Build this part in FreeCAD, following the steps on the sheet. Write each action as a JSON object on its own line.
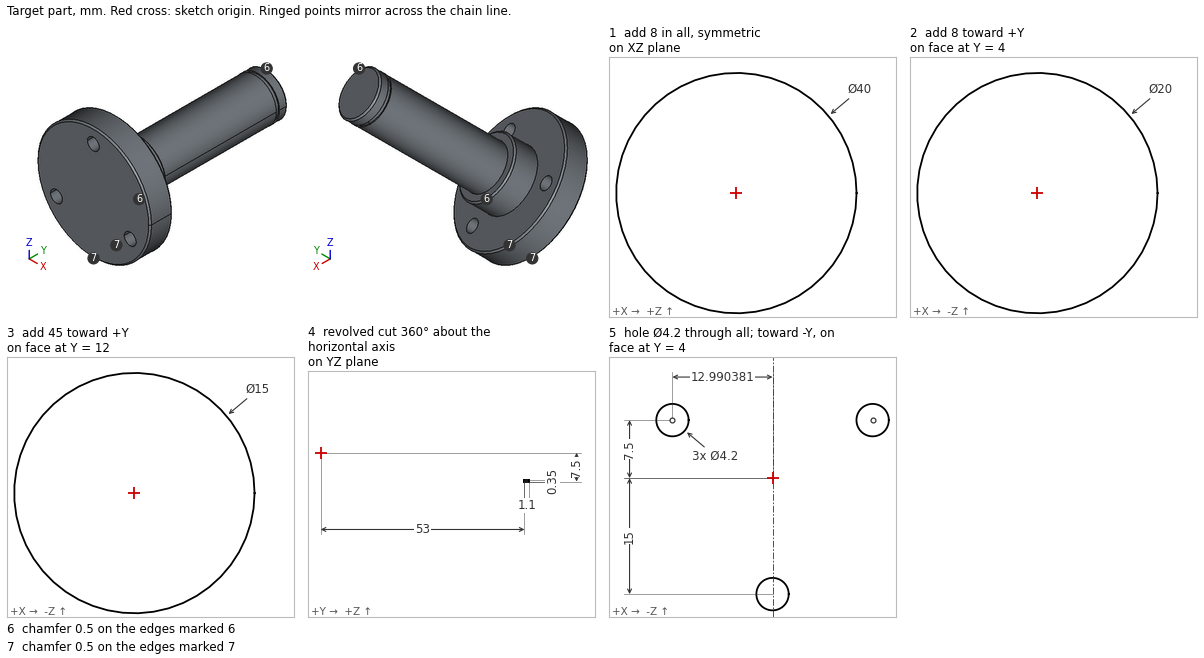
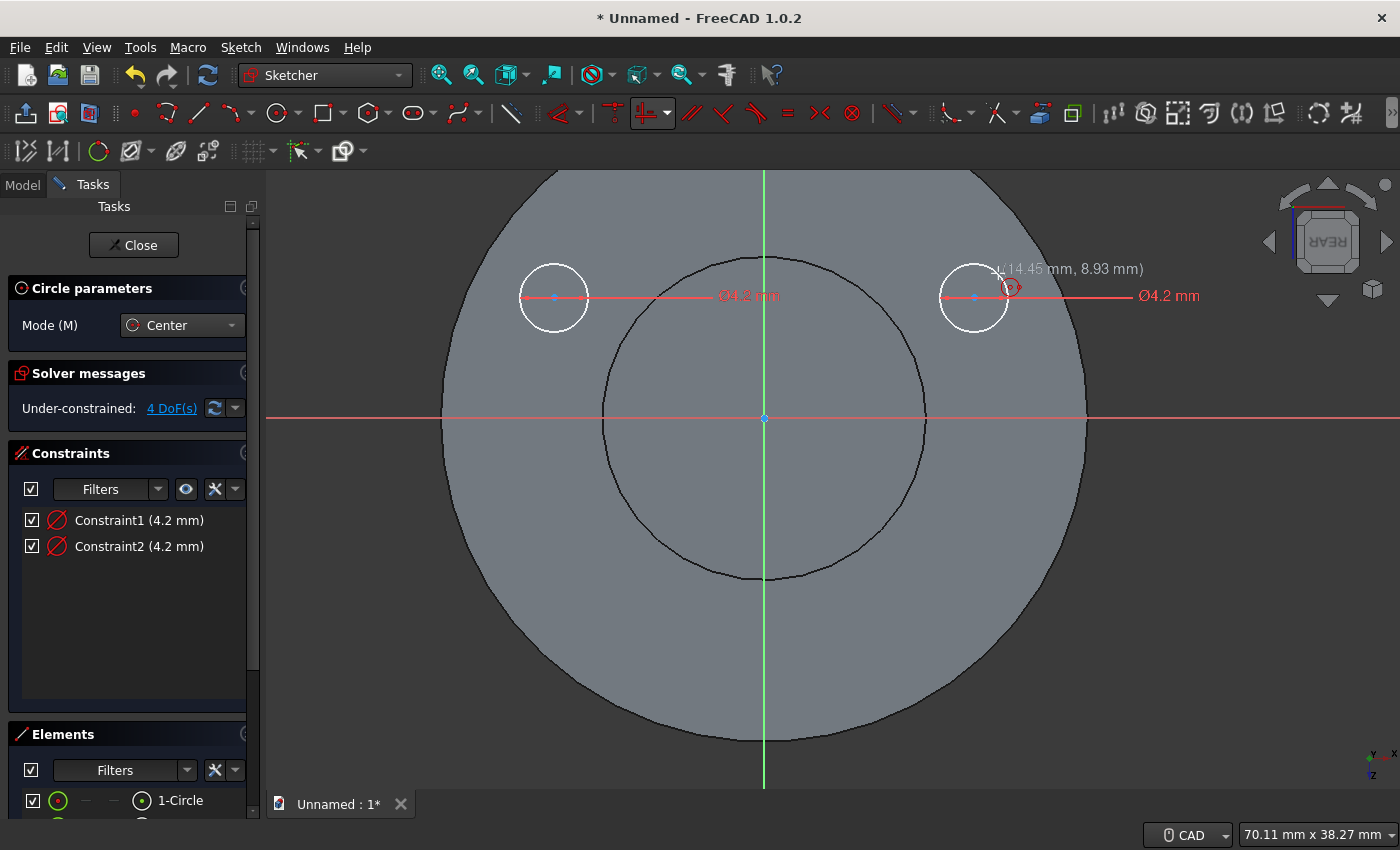
{"action": "left_click", "coordinate": [764, 661]}
{"action": "mouse_move", "coordinate": [788, 637]}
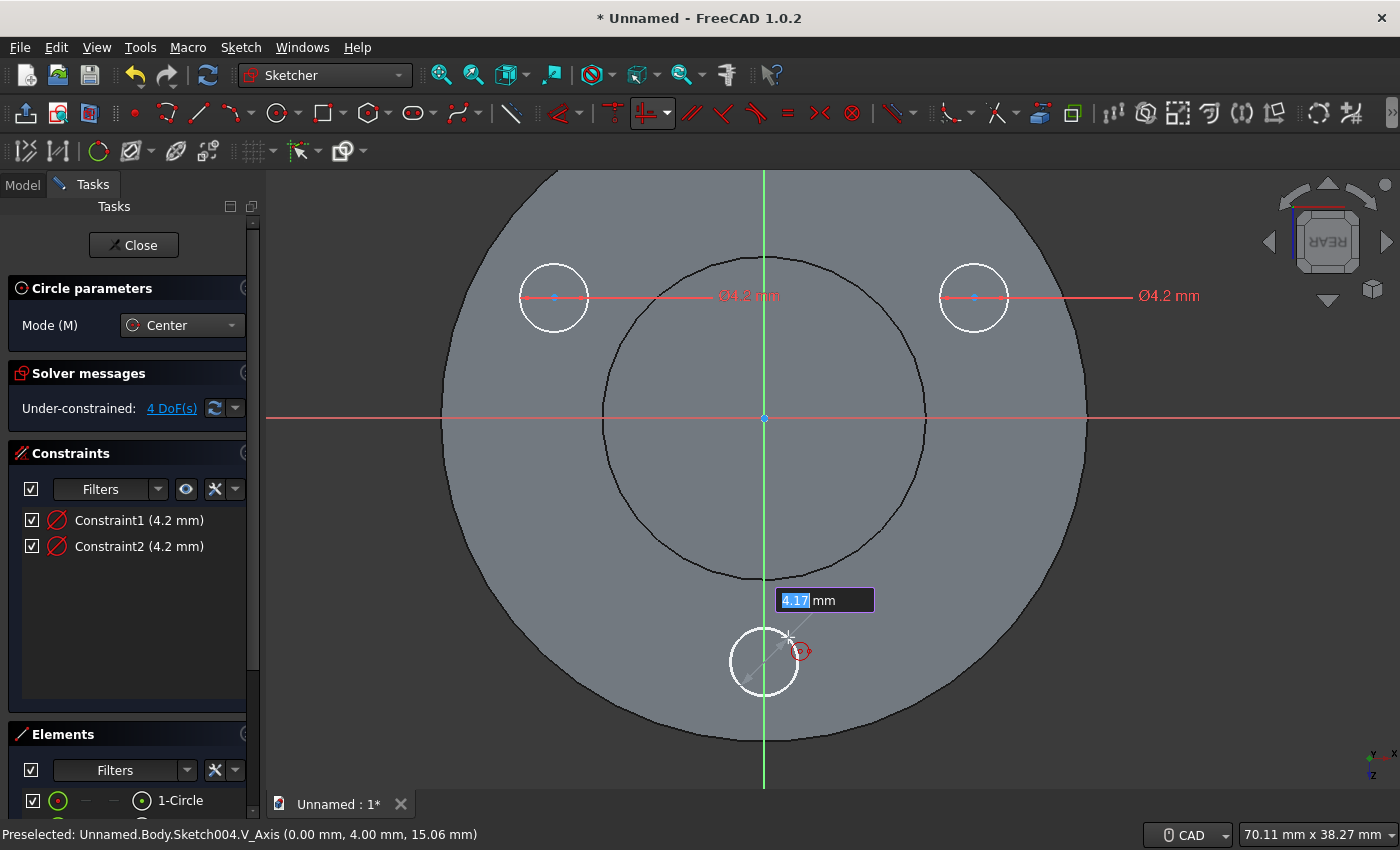
{"action": "type", "text": "4.2"}
{"action": "key", "text": "Return"}
{"action": "key", "text": "Escape"}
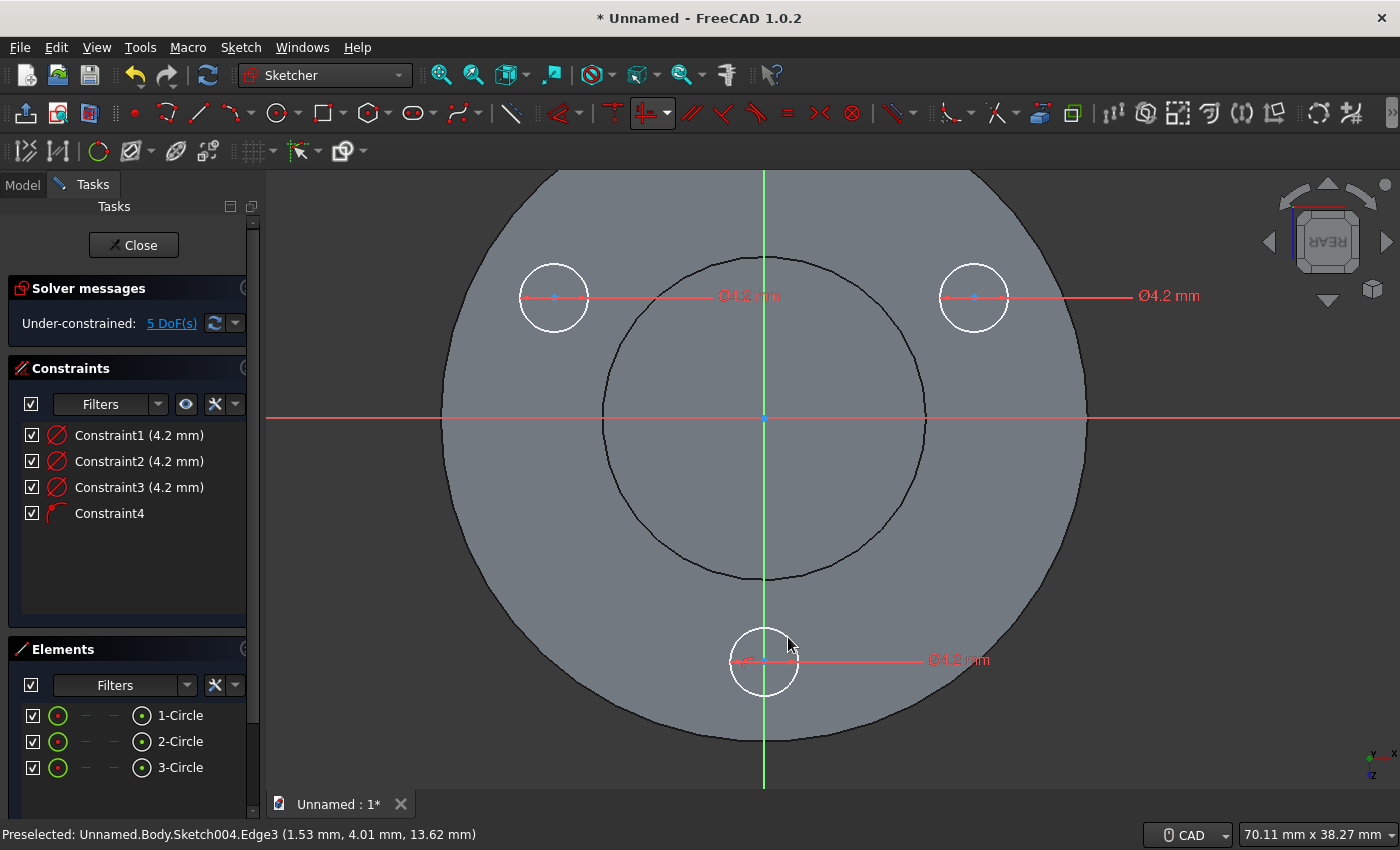
{"action": "left_click", "coordinate": [554, 298]}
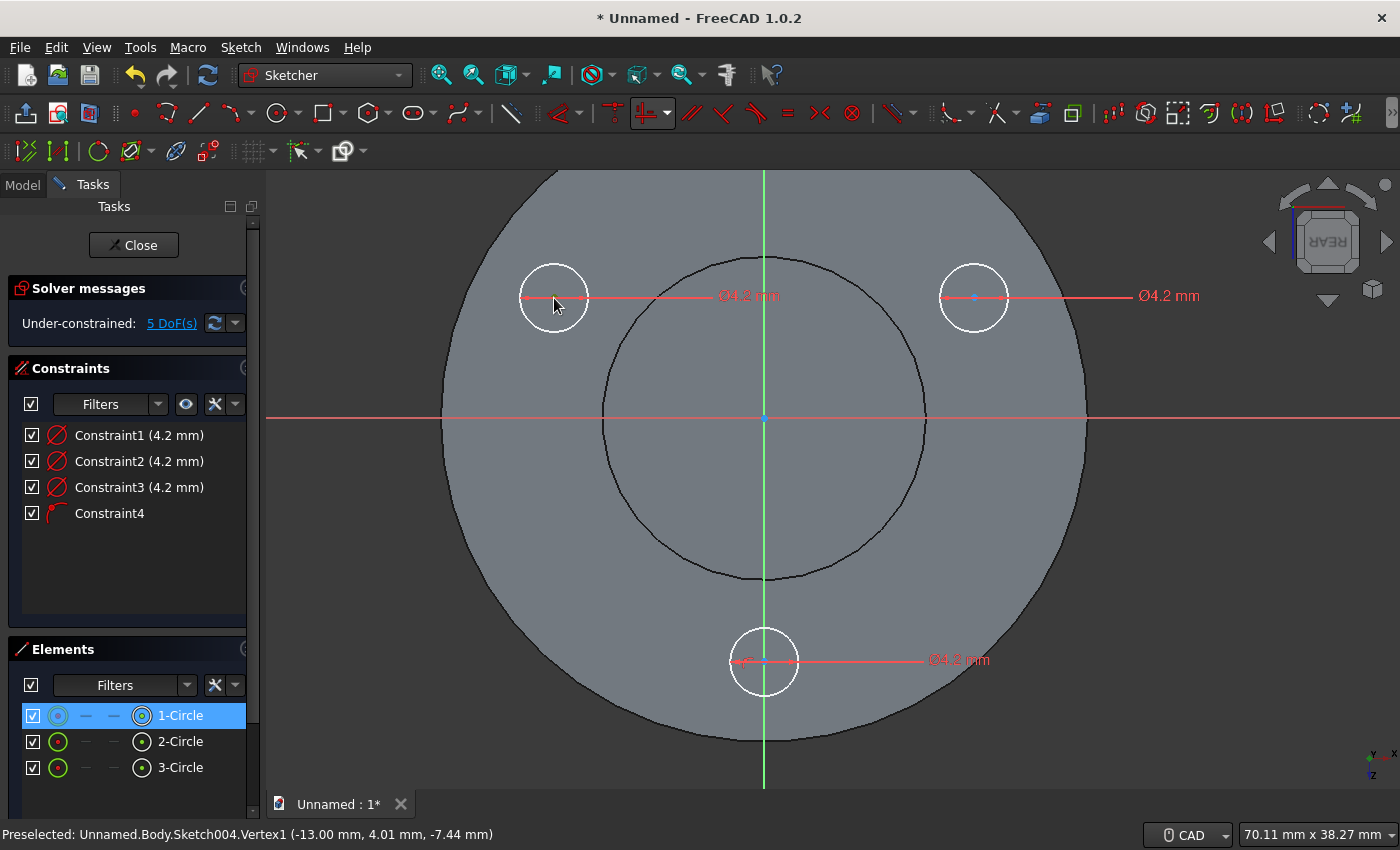
{"action": "left_click", "coordinate": [974, 298]}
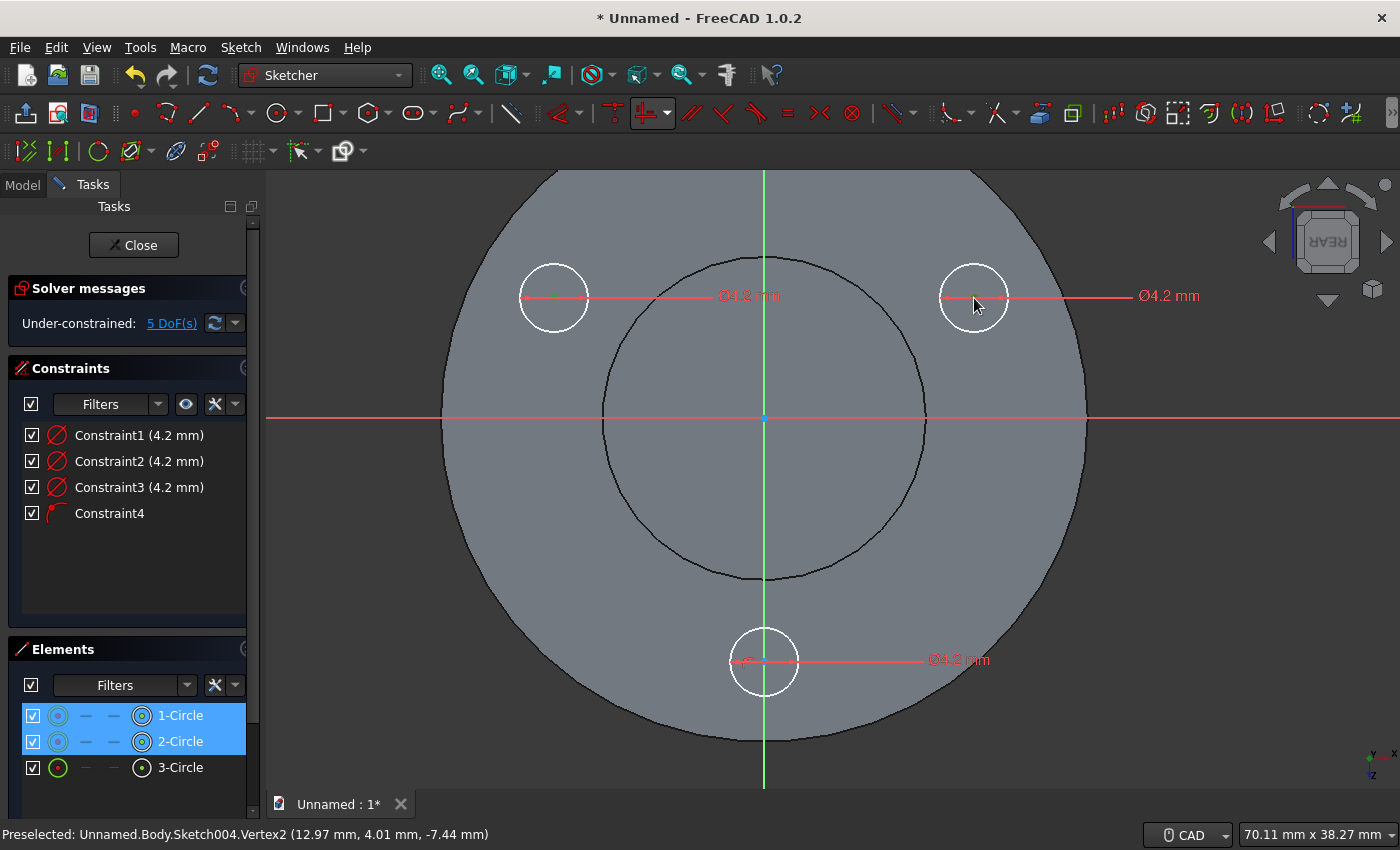
{"action": "left_click", "coordinate": [764, 560]}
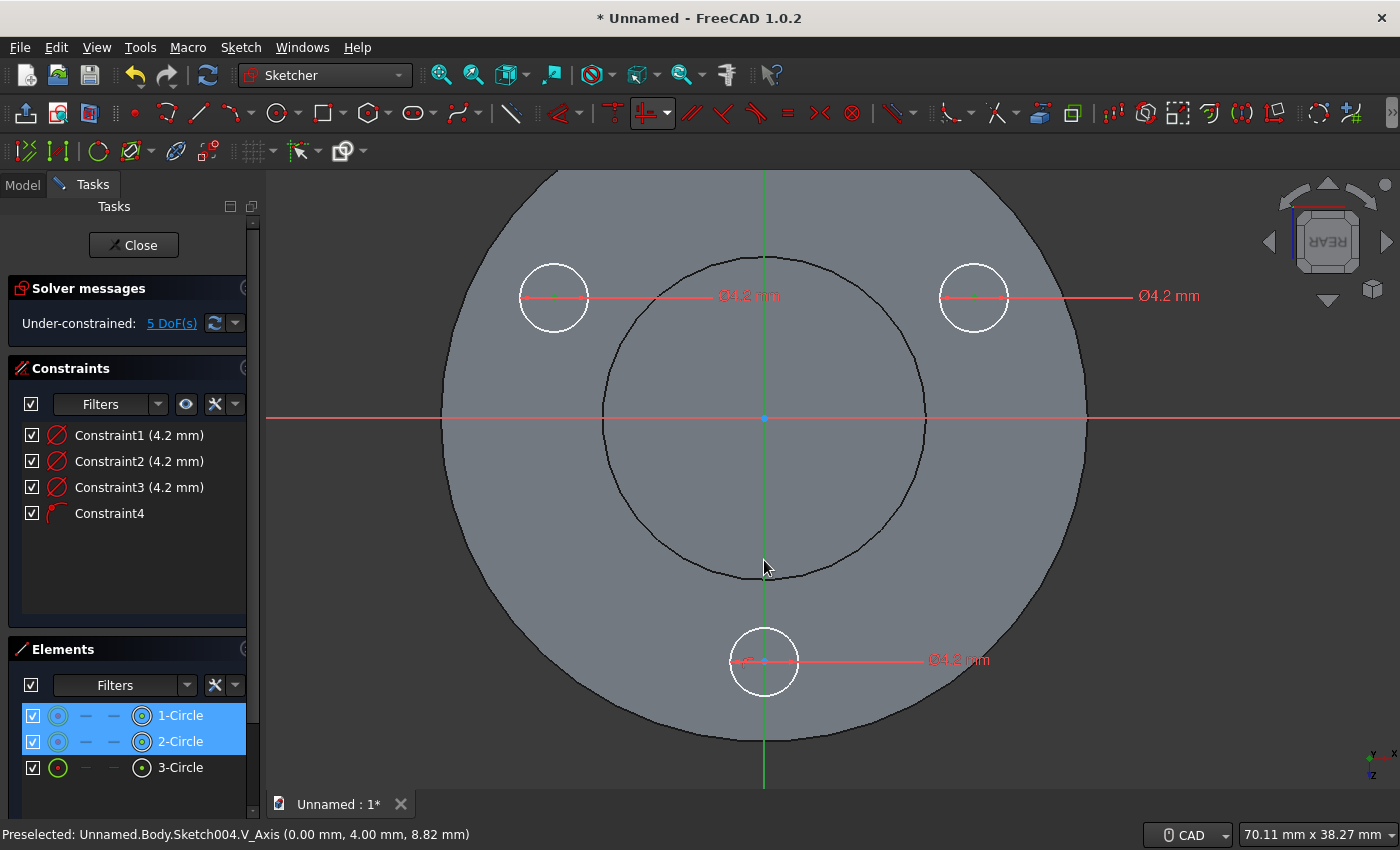
{"action": "left_click", "coordinate": [820, 114]}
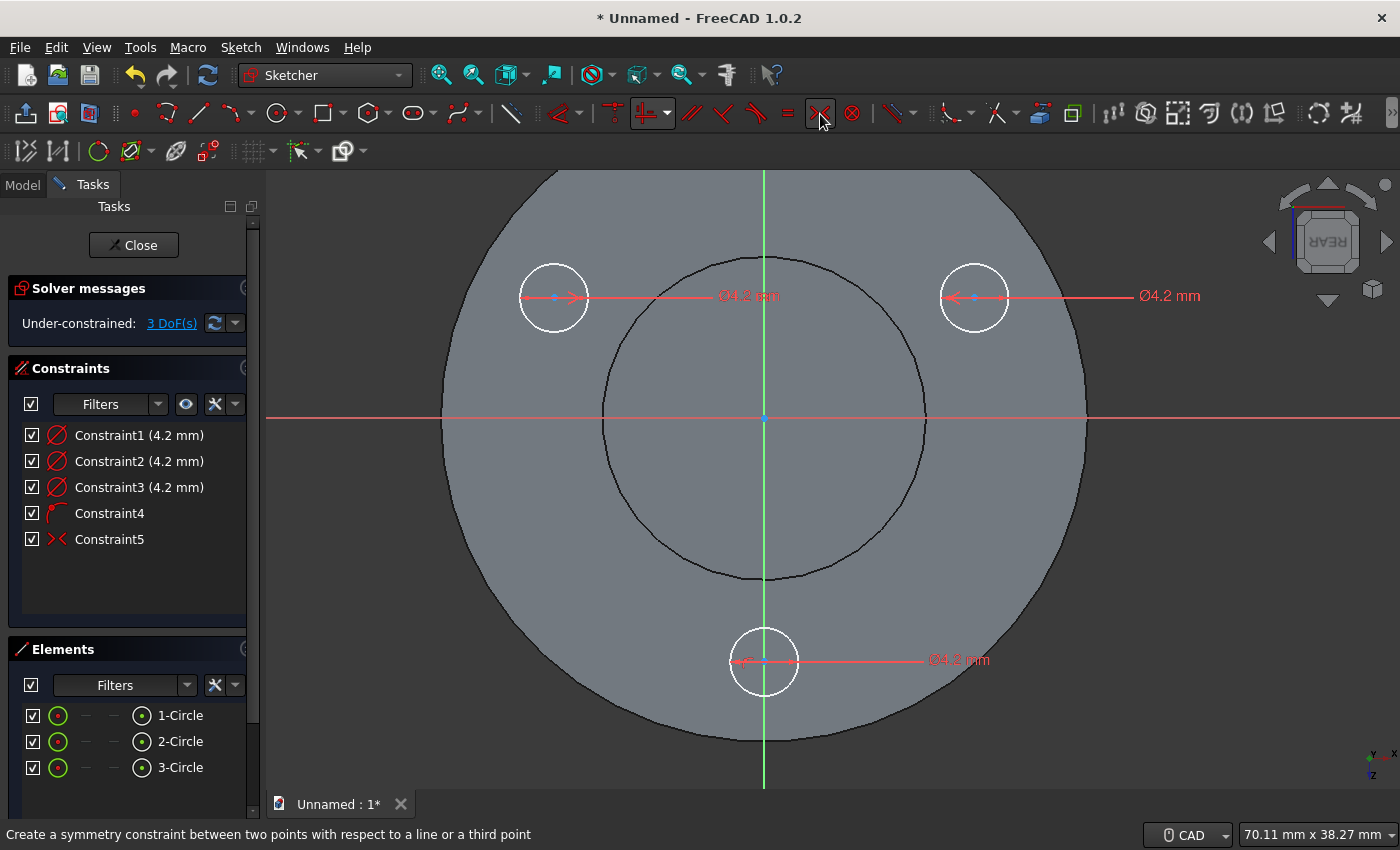
{"action": "left_click", "coordinate": [558, 114]}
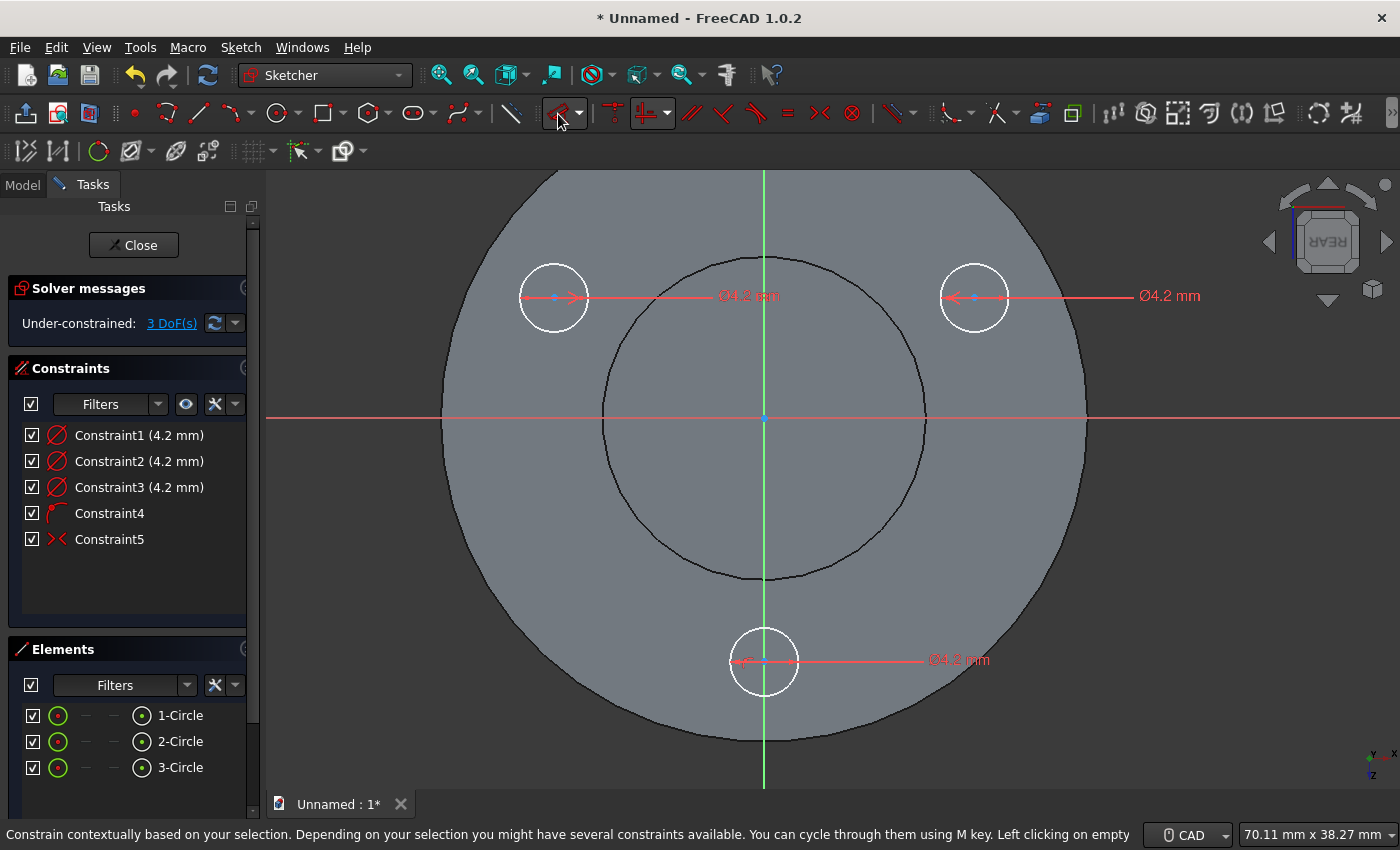
{"action": "left_click", "coordinate": [764, 662]}
{"action": "left_click", "coordinate": [798, 540]}